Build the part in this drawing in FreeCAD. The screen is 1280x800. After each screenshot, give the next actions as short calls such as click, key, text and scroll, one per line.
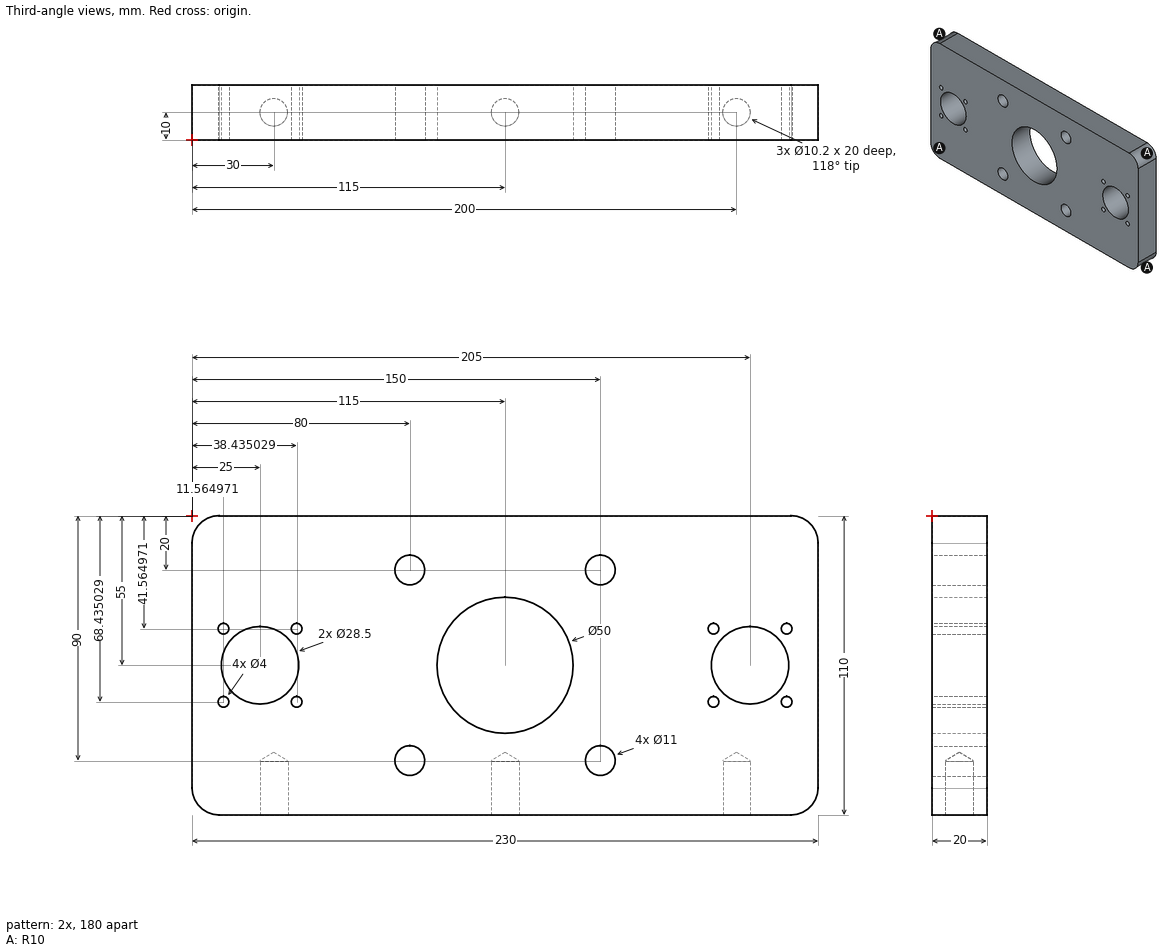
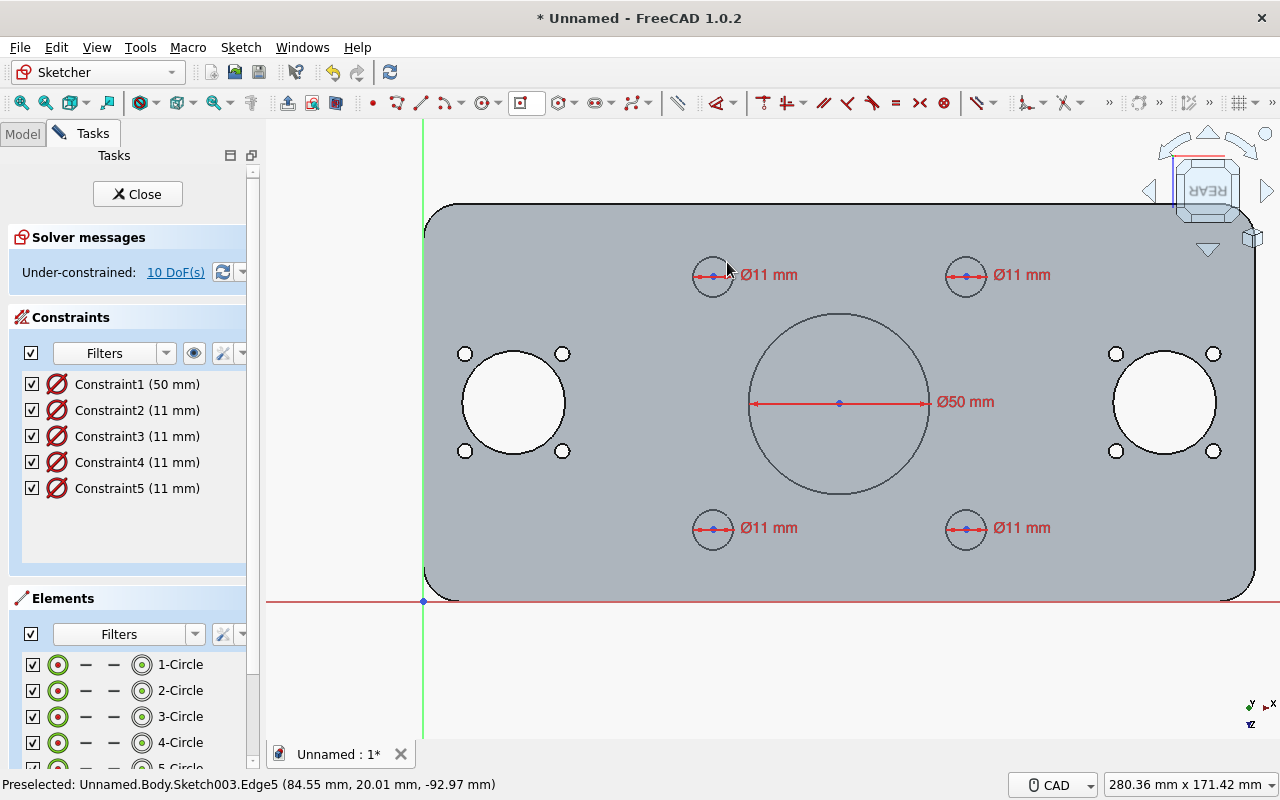
click(716, 104)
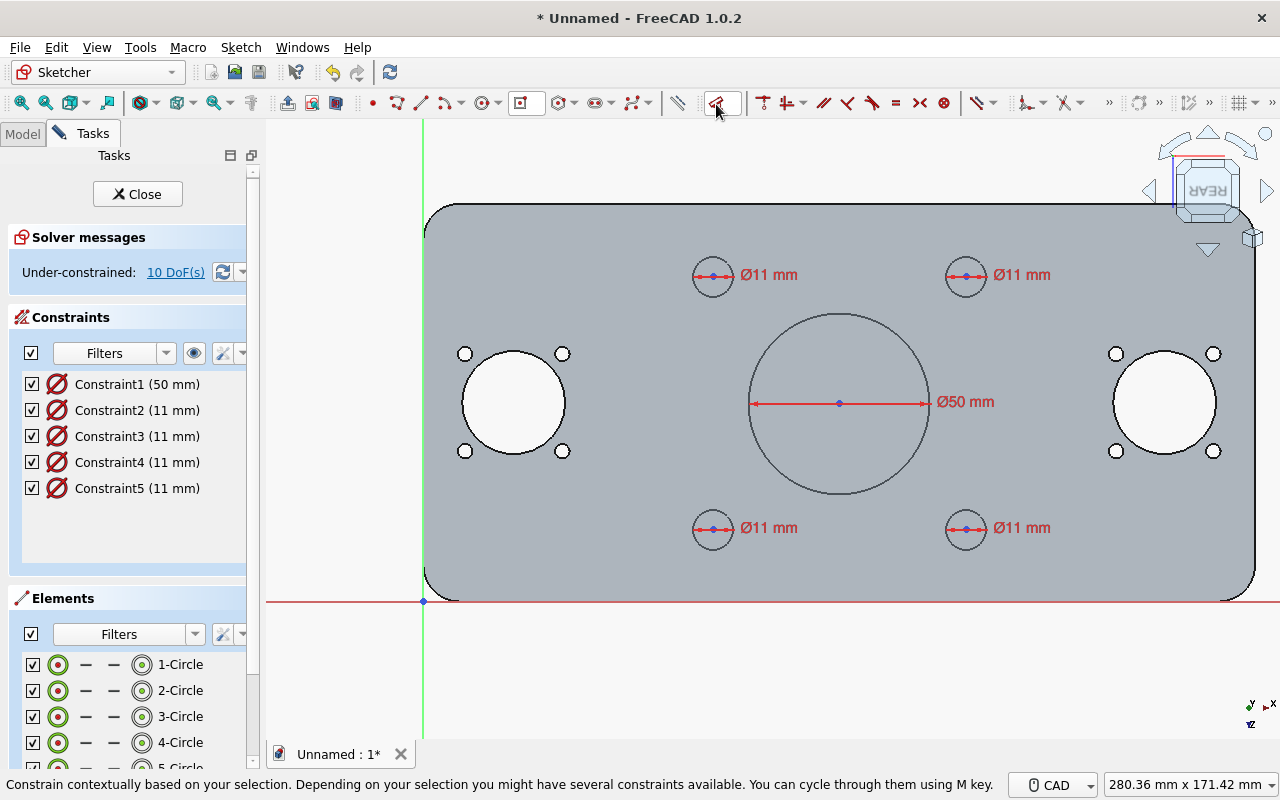
click(839, 404)
click(389, 503)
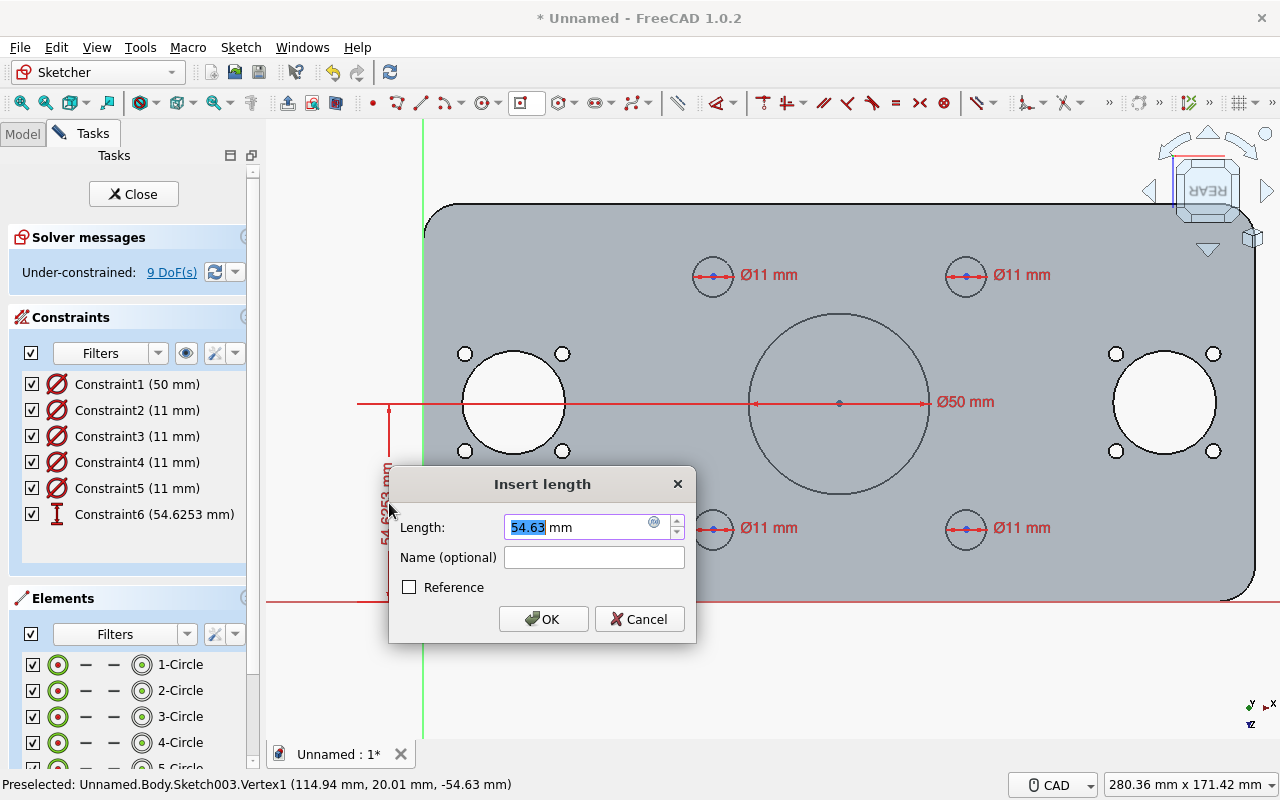
text(55)
key(Return)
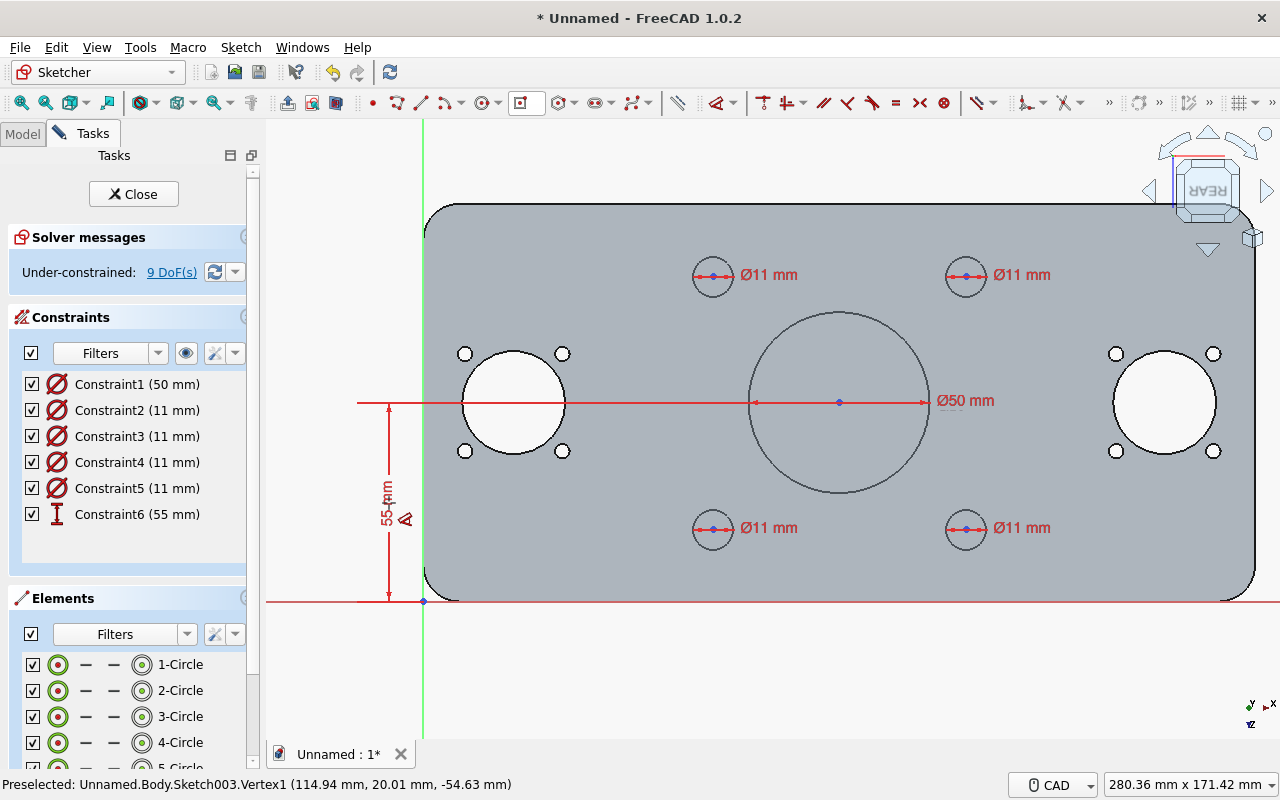
click(966, 277)
click(389, 439)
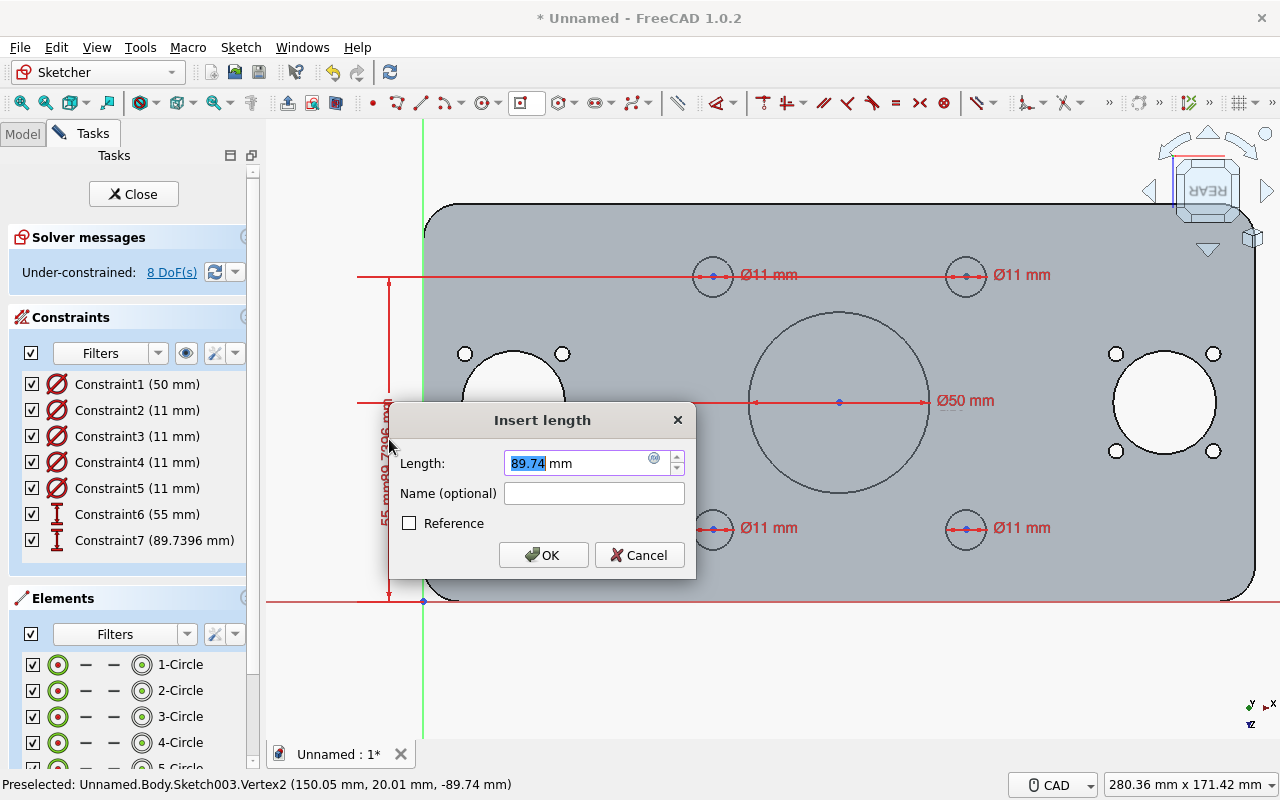
text(90)
key(Return)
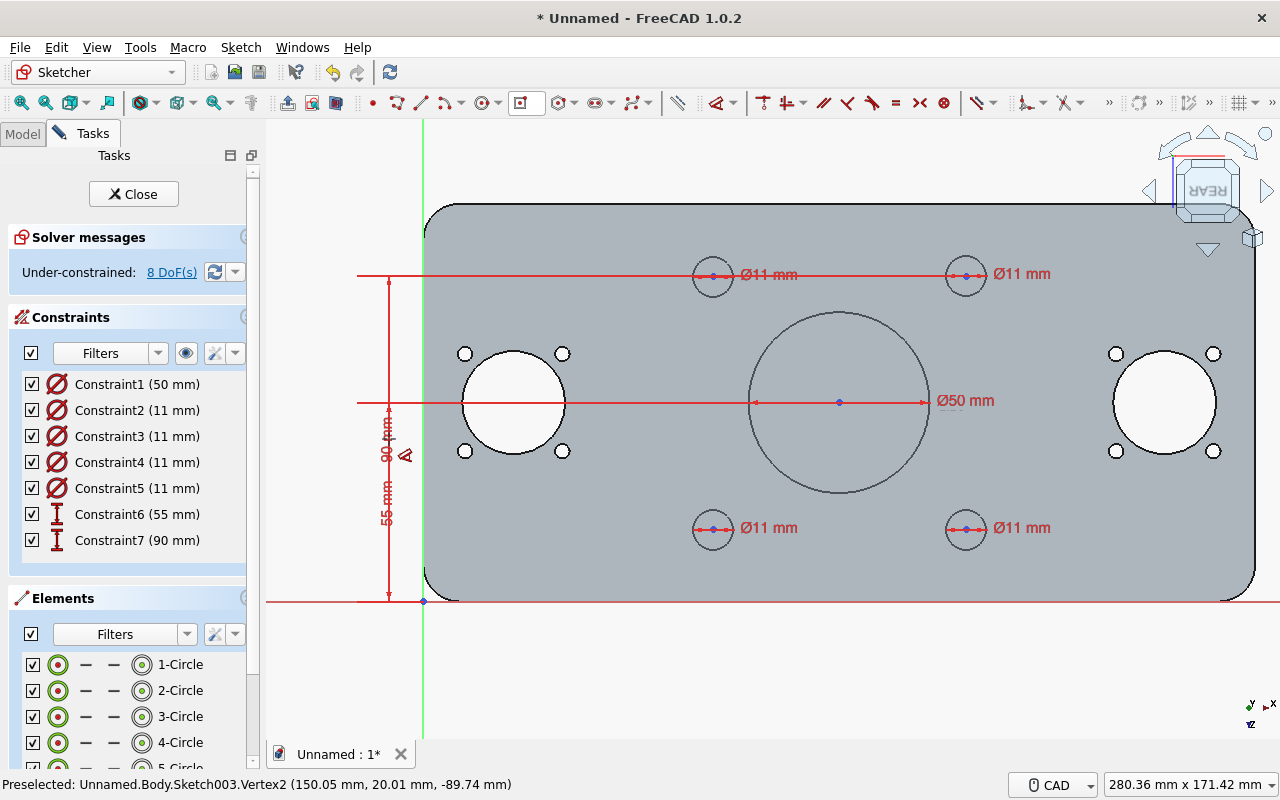
click(966, 530)
click(389, 566)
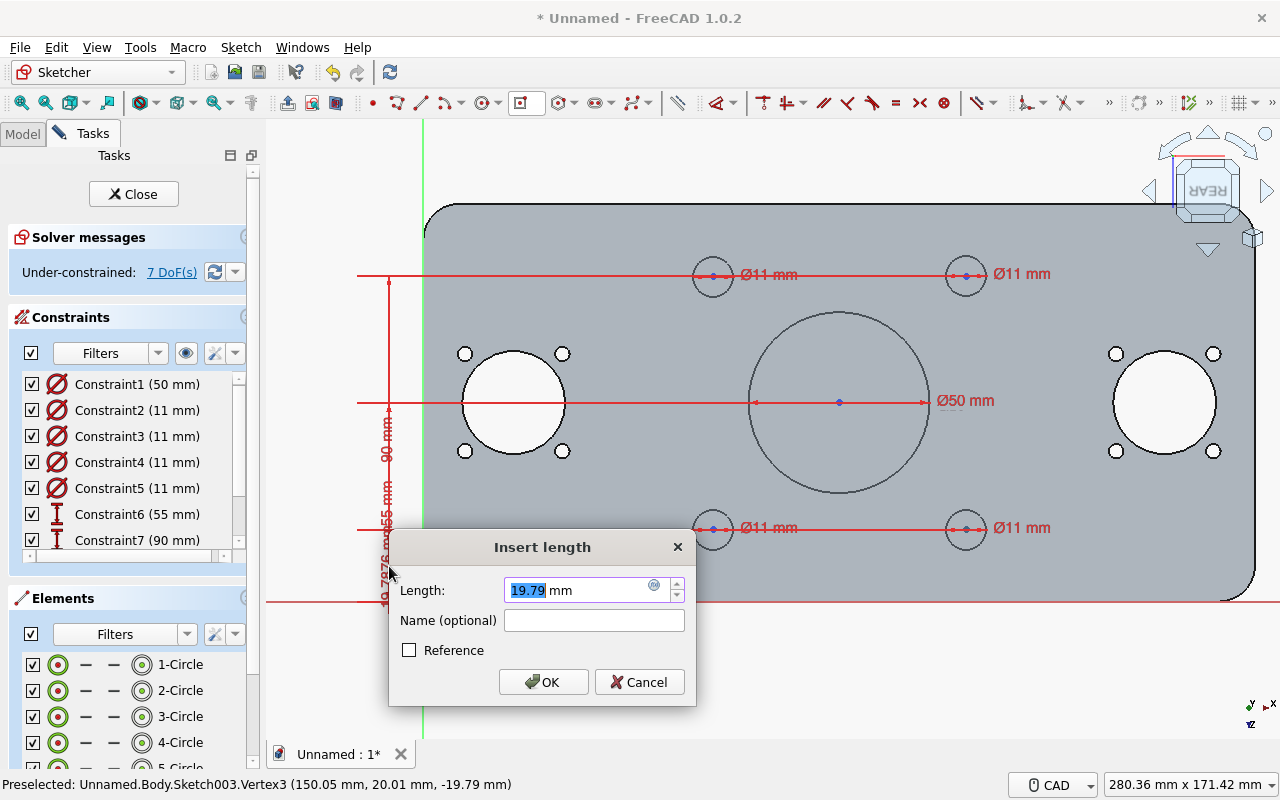
text(20)
key(Return)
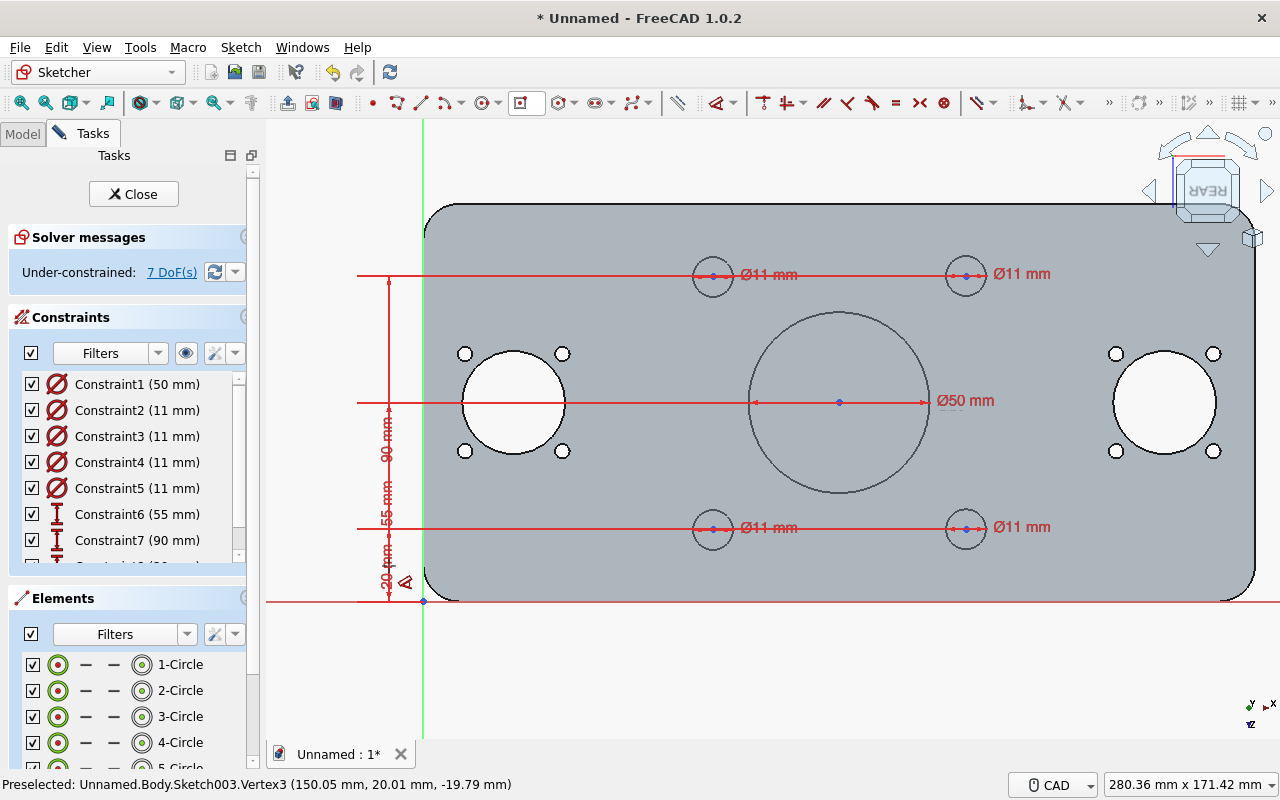
click(713, 530)
click(568, 636)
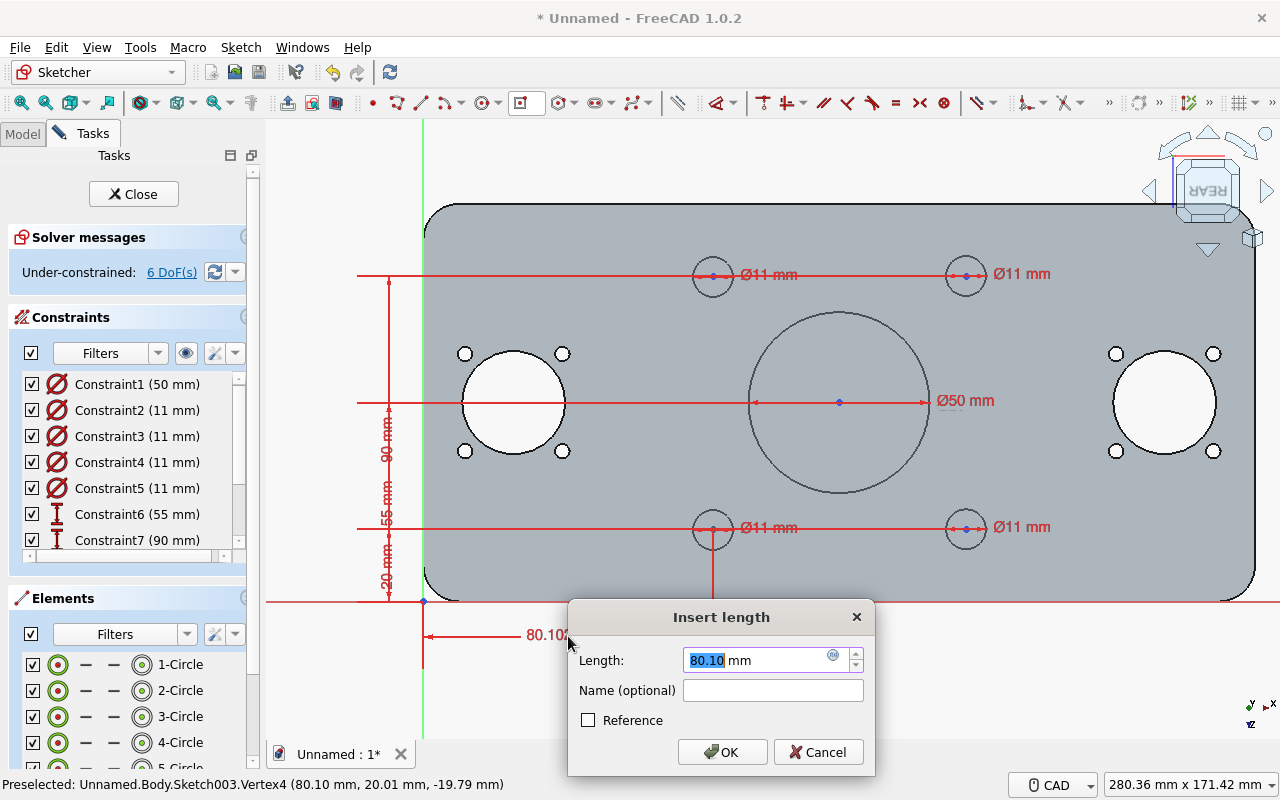
text(80)
key(Return)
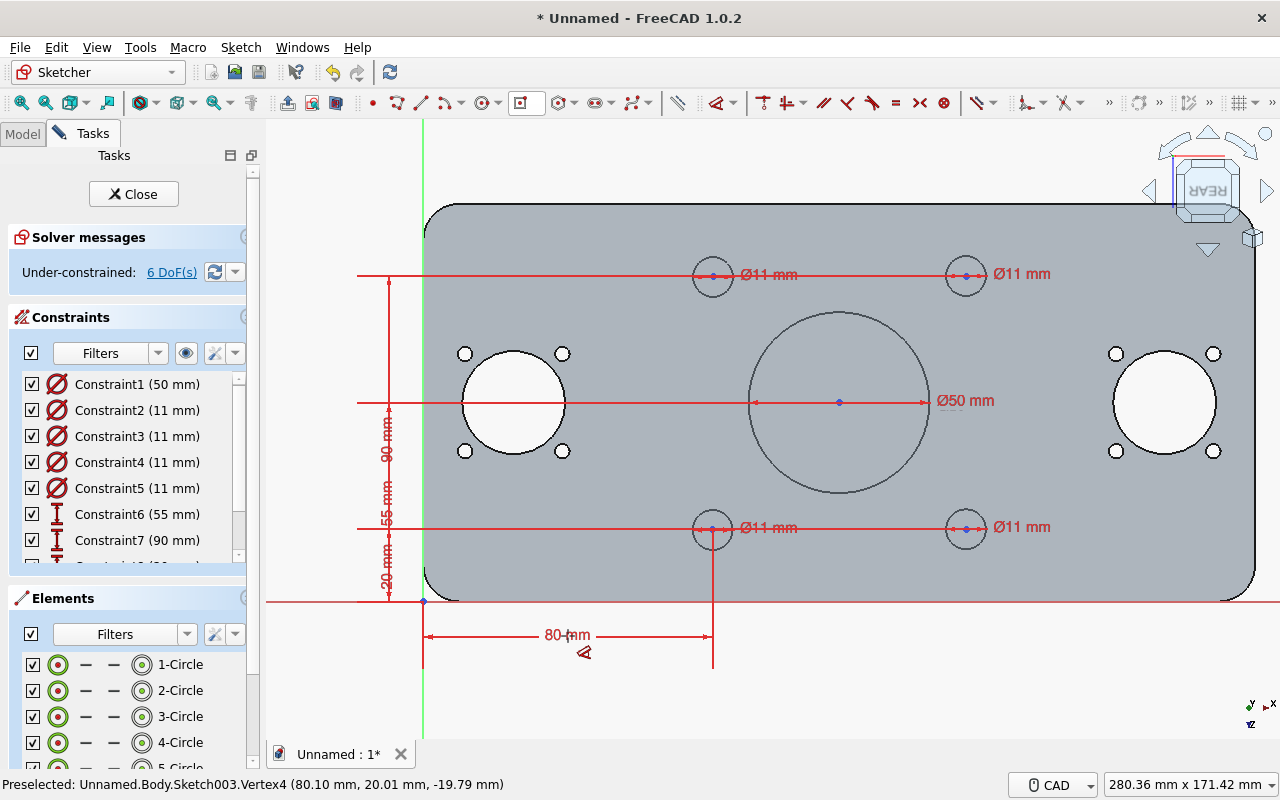
click(713, 530)
click(389, 541)